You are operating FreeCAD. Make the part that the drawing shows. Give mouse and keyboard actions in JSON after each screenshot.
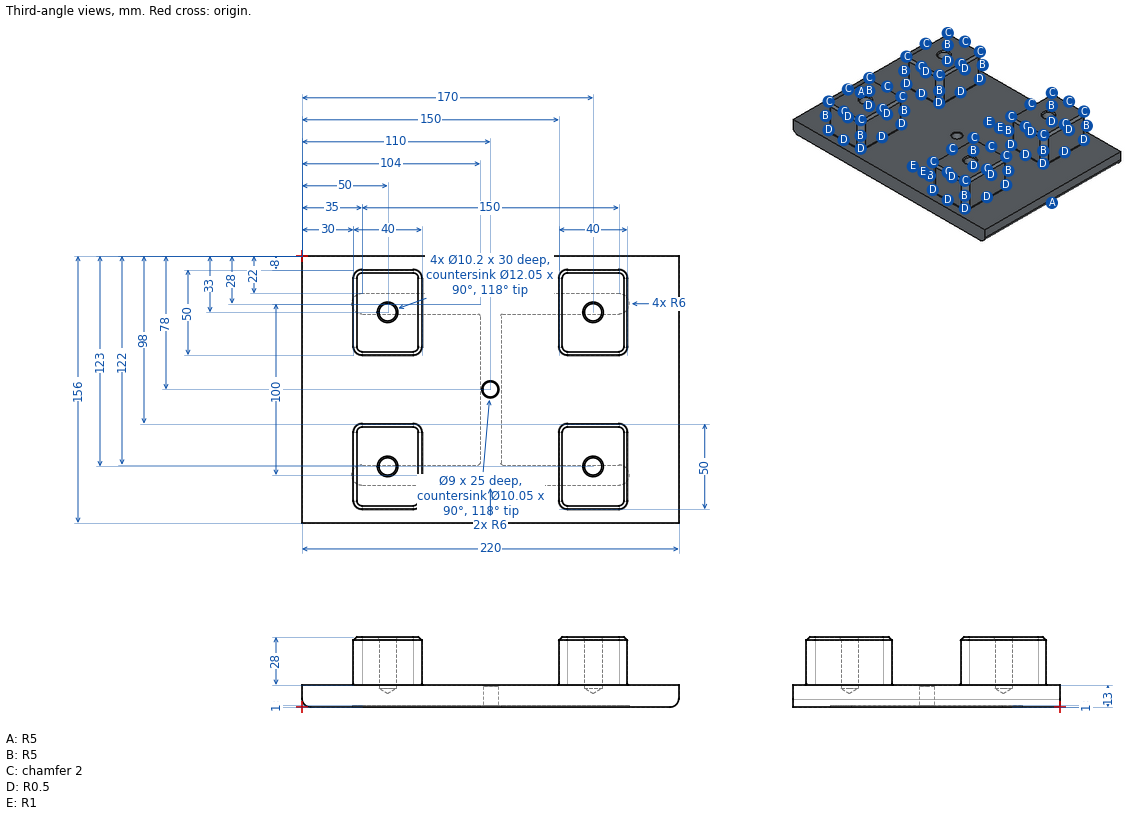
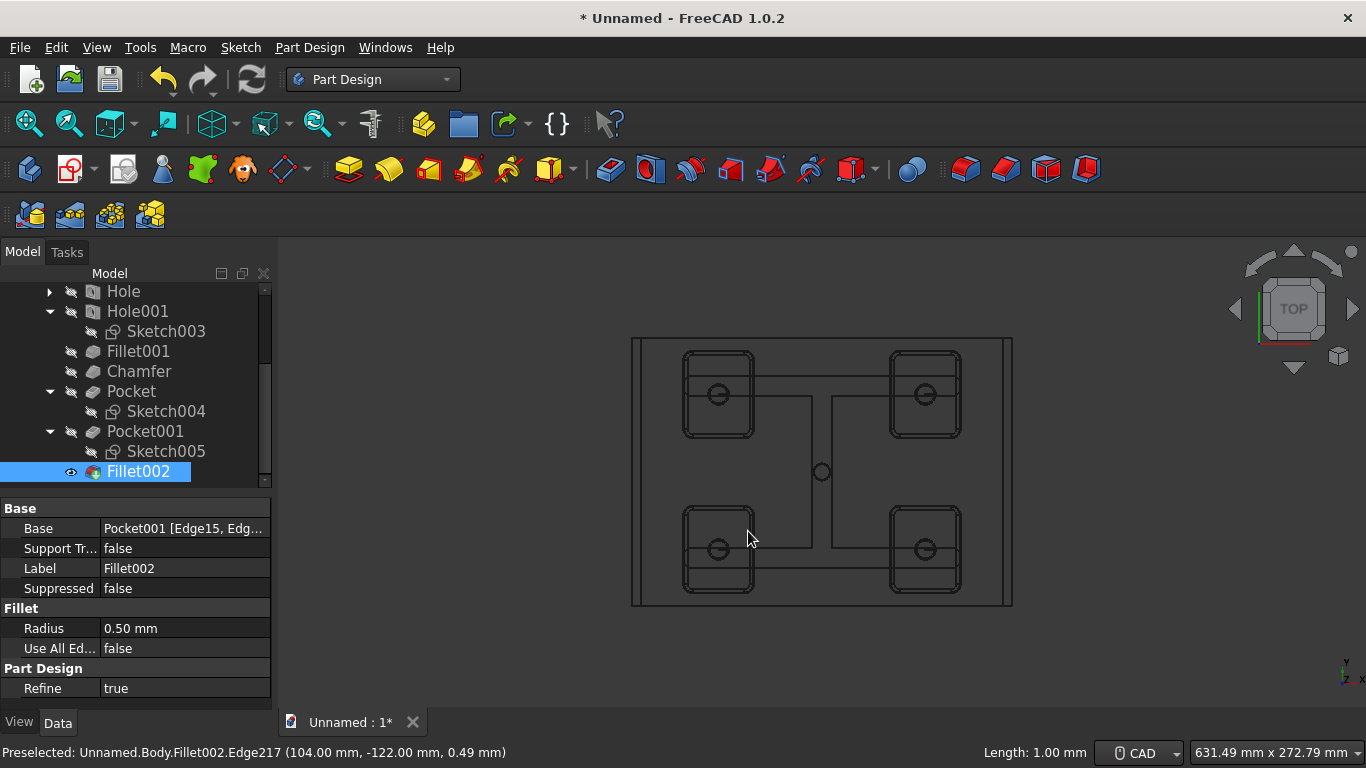
{"action": "scroll", "coordinate": [812, 395], "scroll_direction": "up", "scroll_amount": 15}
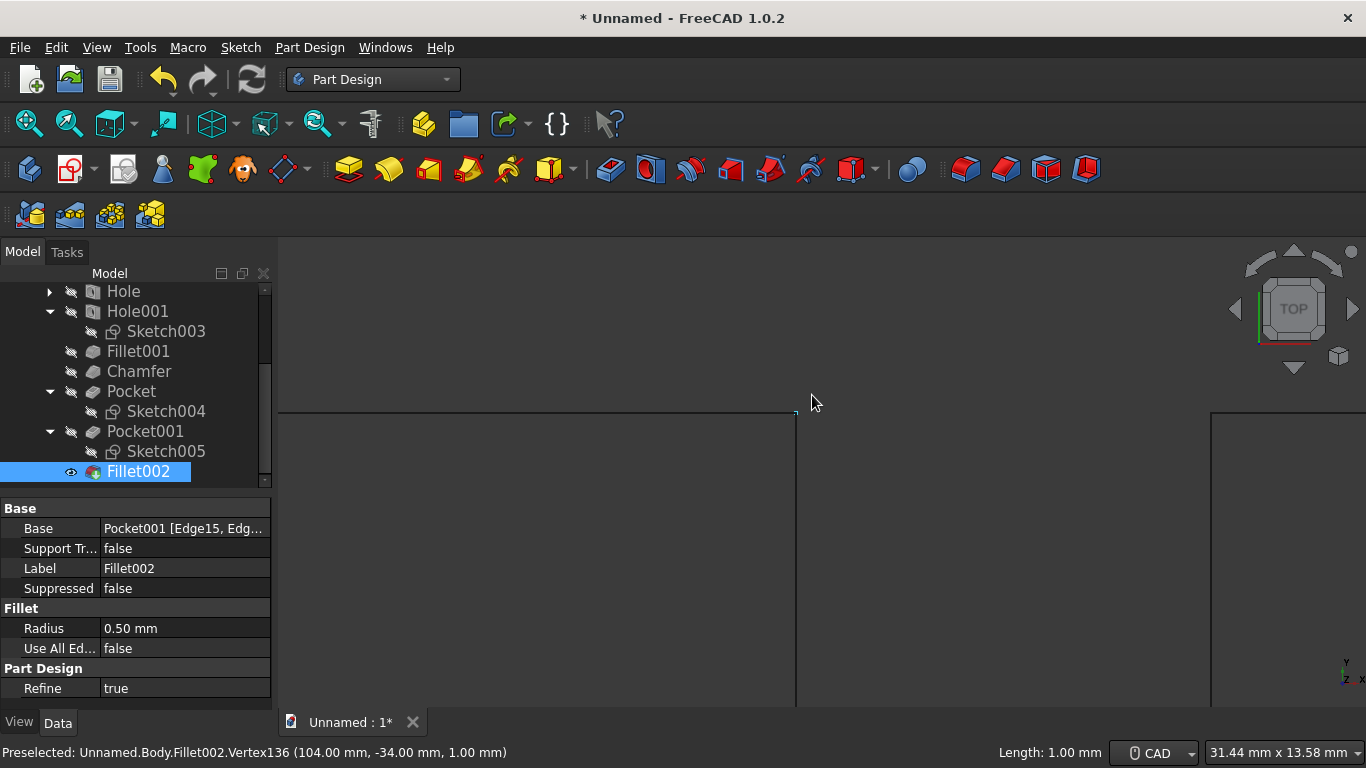
{"action": "key", "text": "v f"}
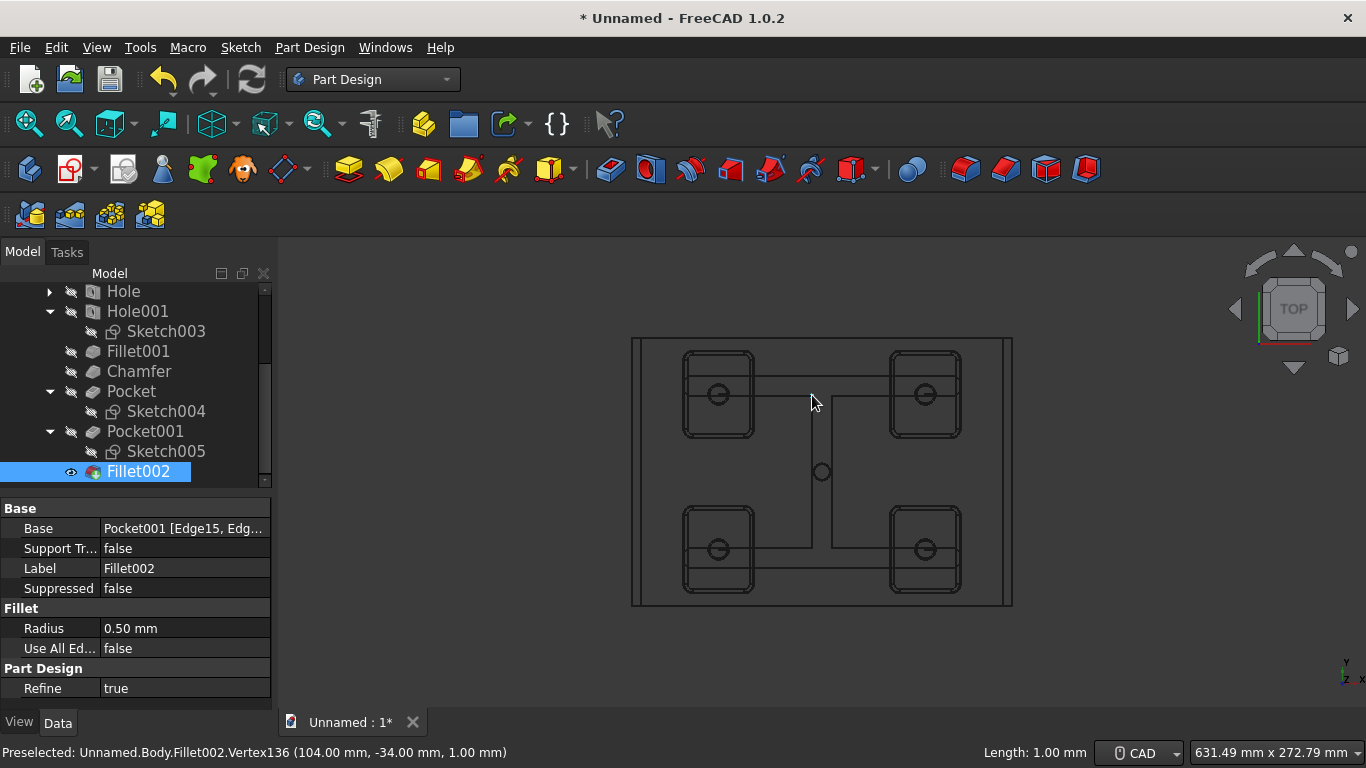
{"action": "key", "text": "1"}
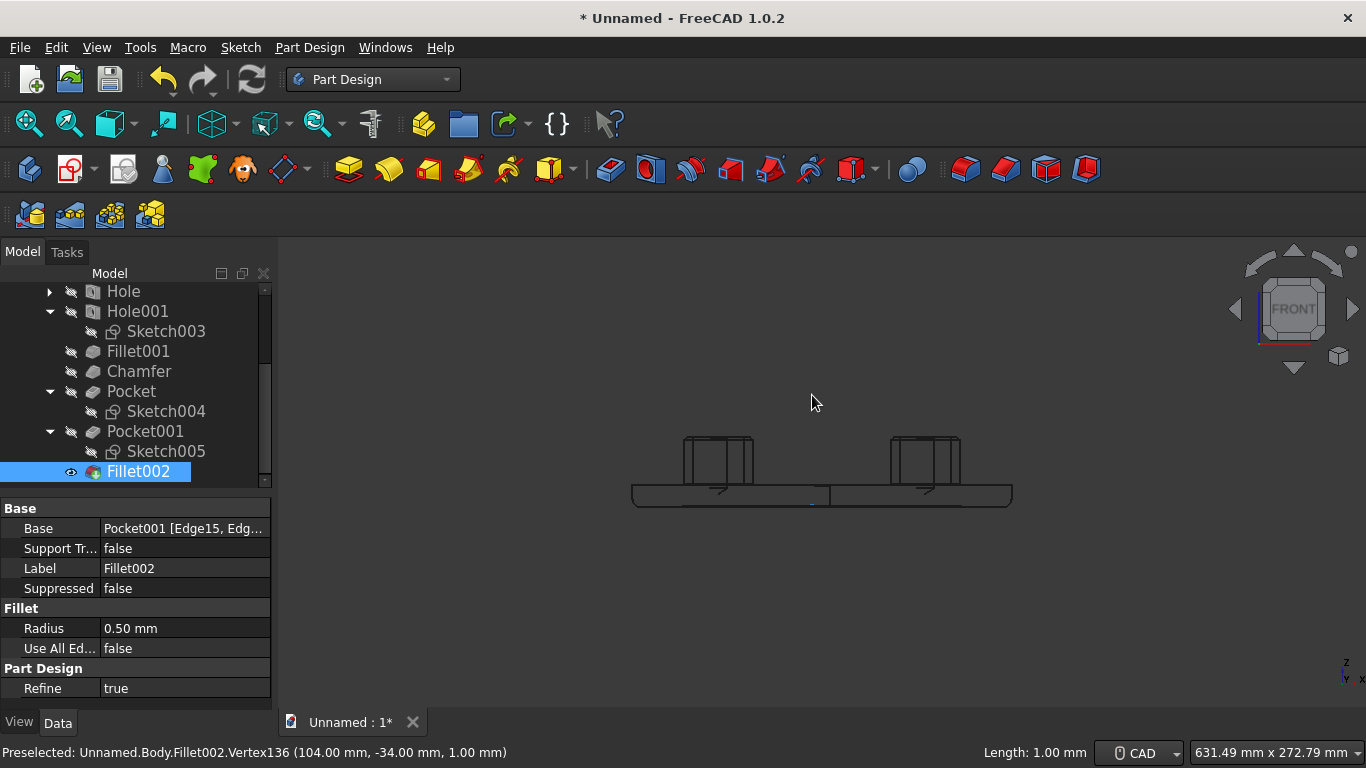
{"action": "key", "text": "v f"}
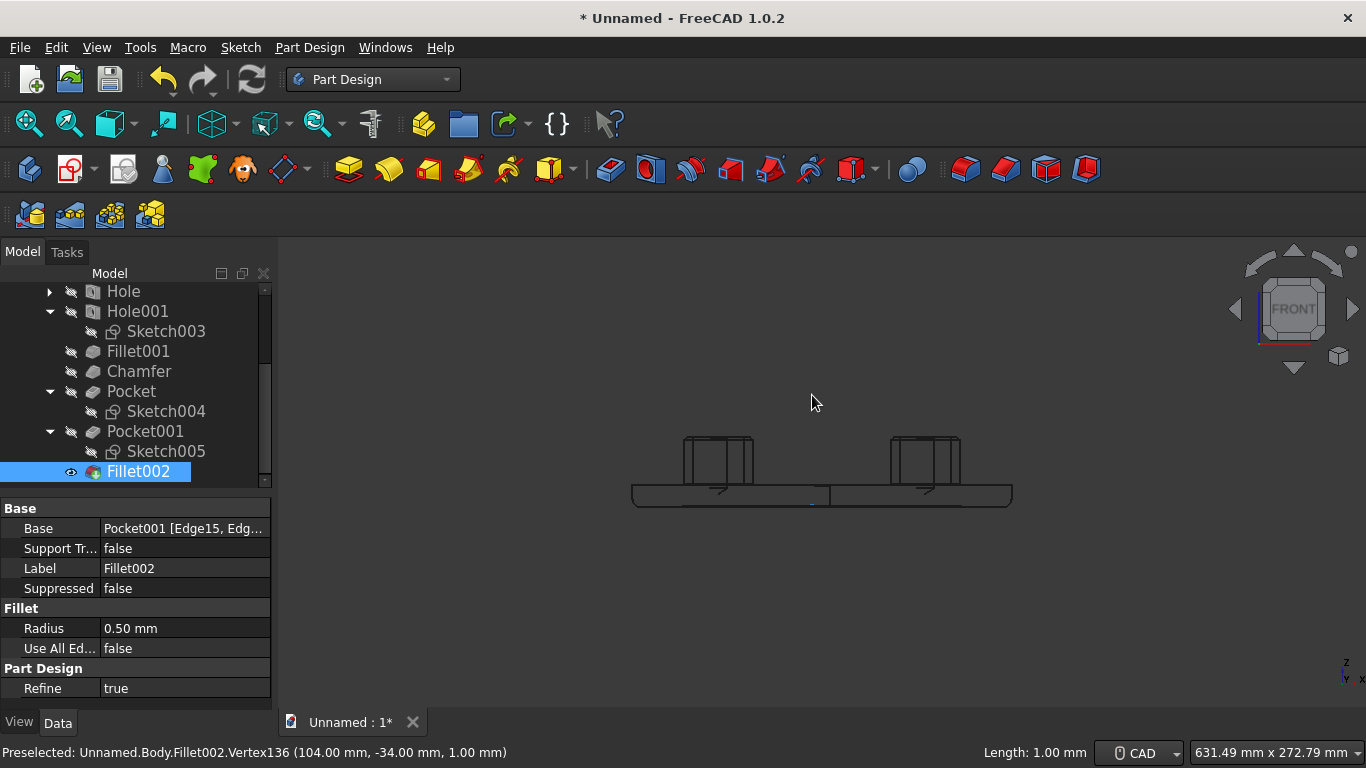
{"action": "scroll", "coordinate": [812, 505], "scroll_direction": "up", "scroll_amount": 15}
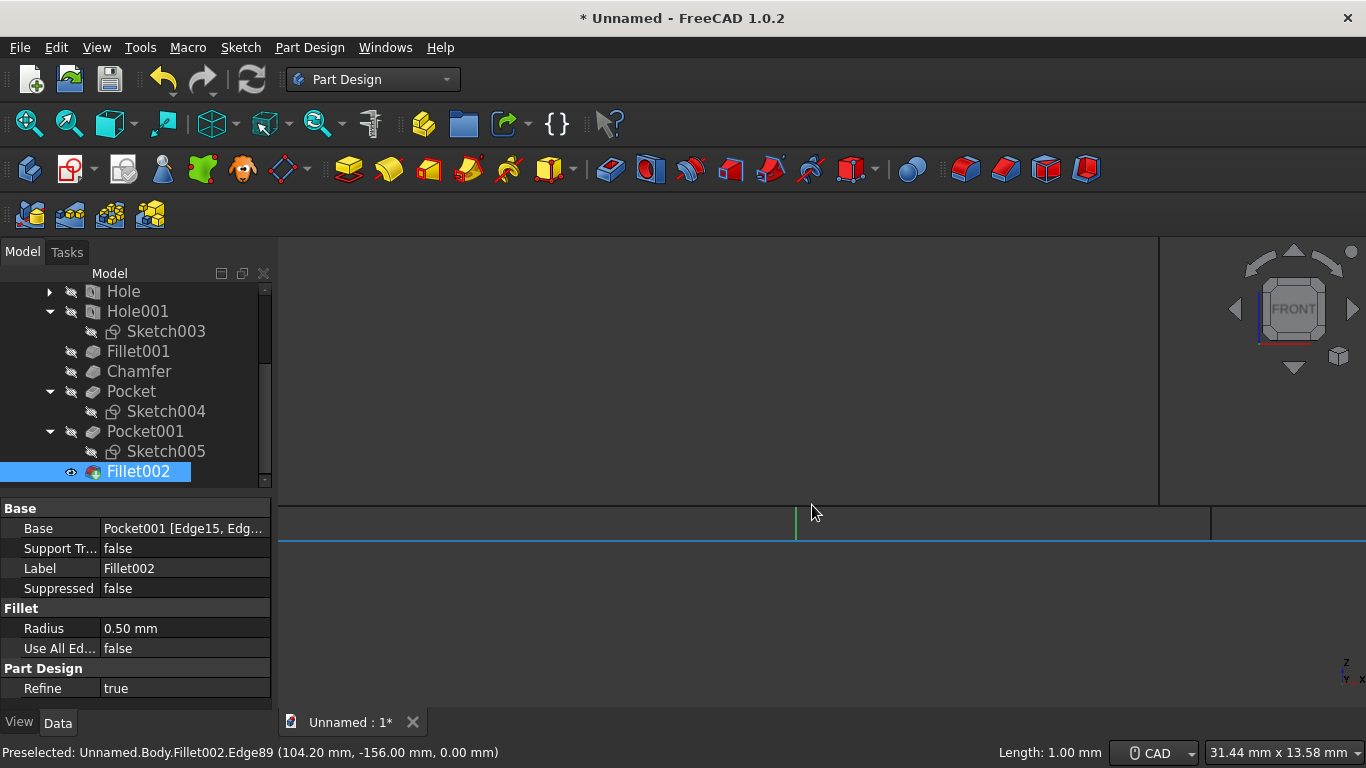
{"action": "left_click", "coordinate": [1211, 522], "text": "ctrl"}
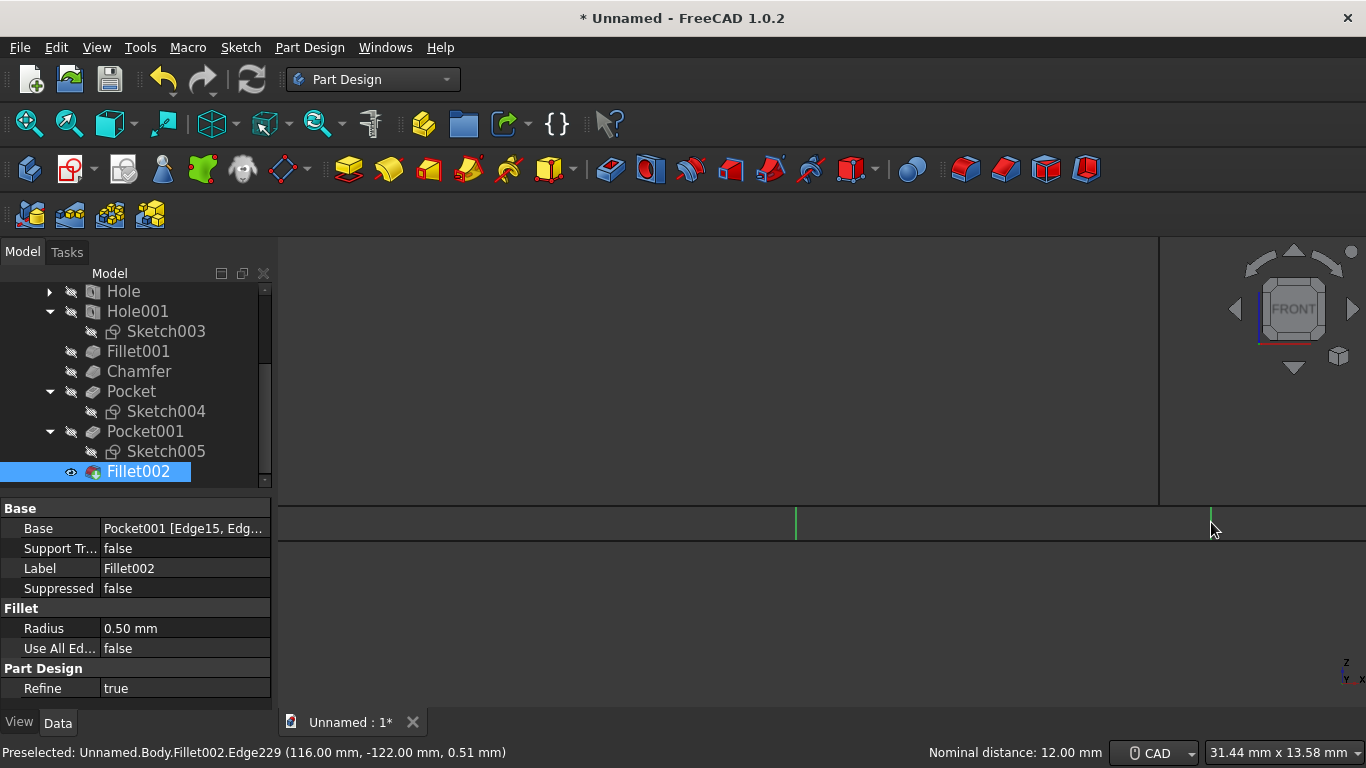
{"action": "left_click", "coordinate": [30, 124]}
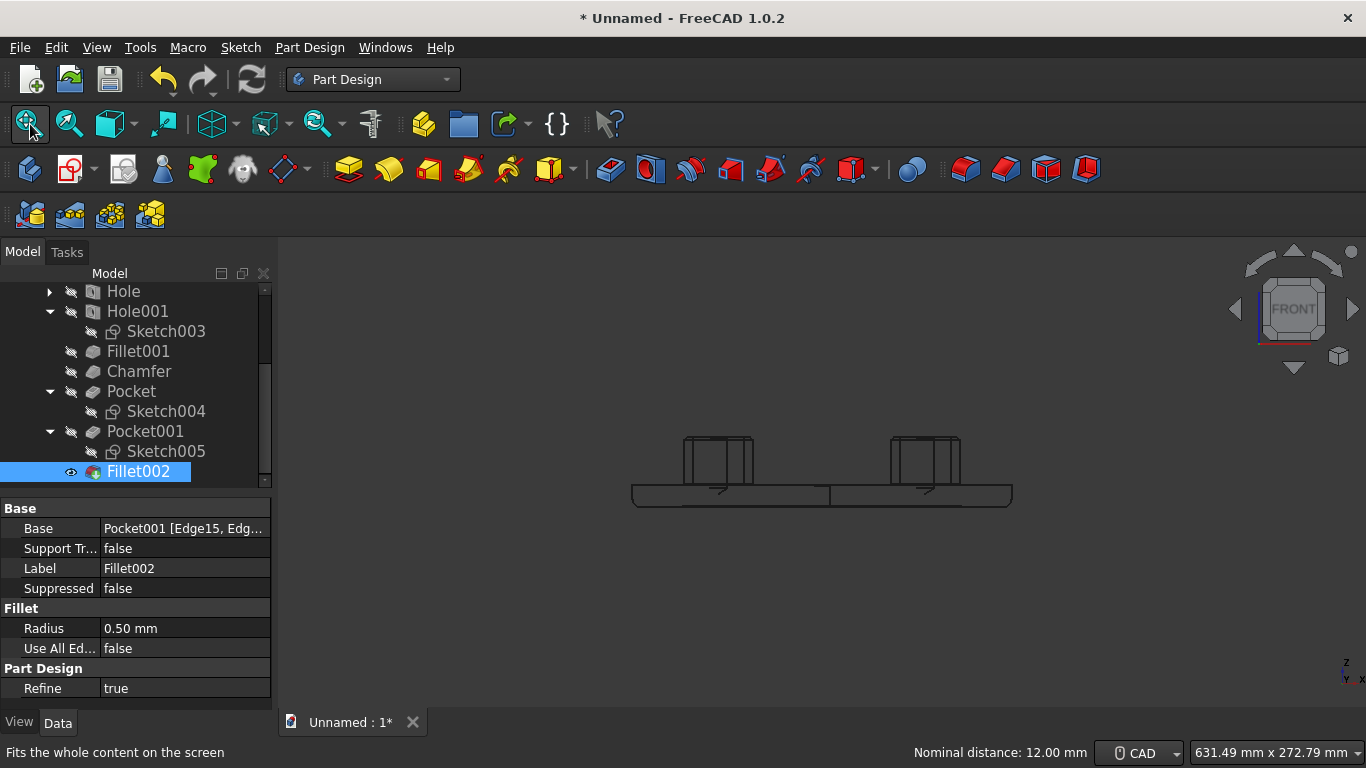
{"action": "key", "text": "3"}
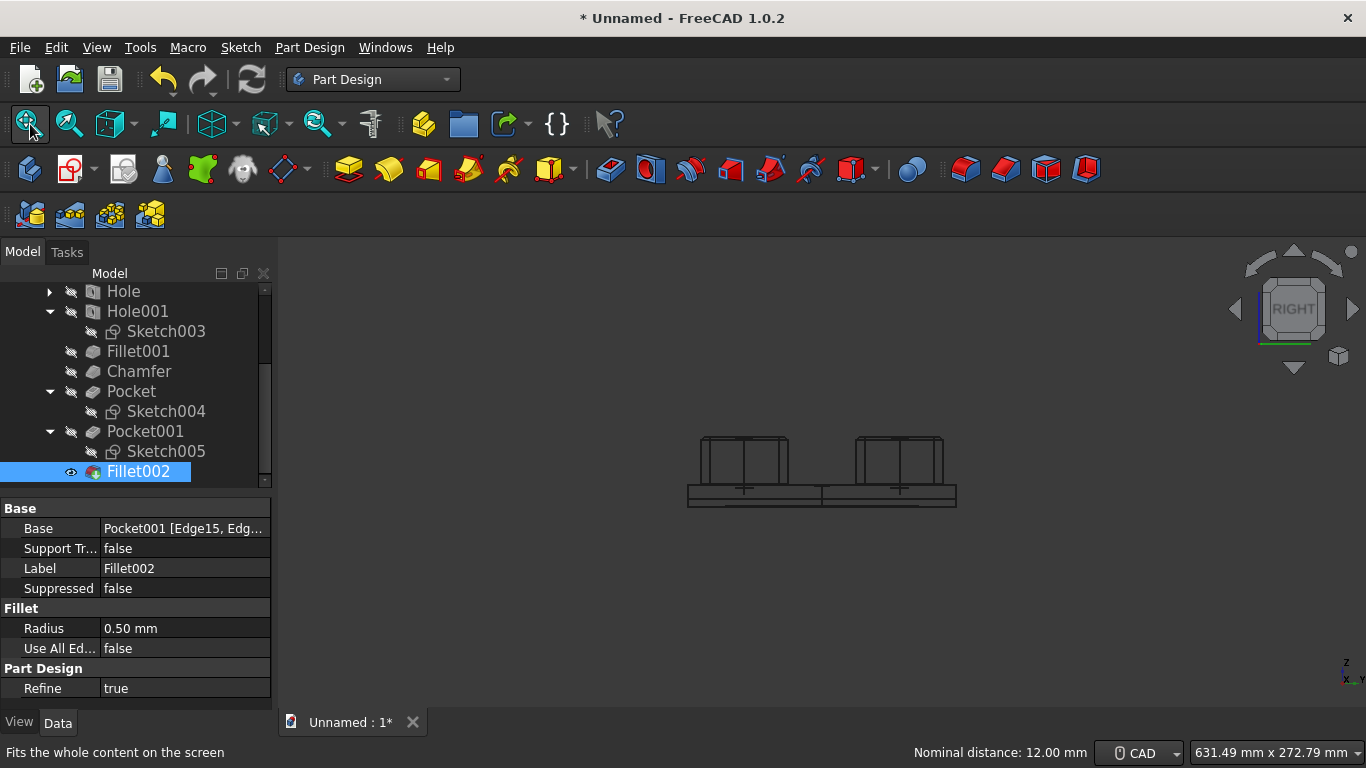
{"action": "key", "text": "v f"}